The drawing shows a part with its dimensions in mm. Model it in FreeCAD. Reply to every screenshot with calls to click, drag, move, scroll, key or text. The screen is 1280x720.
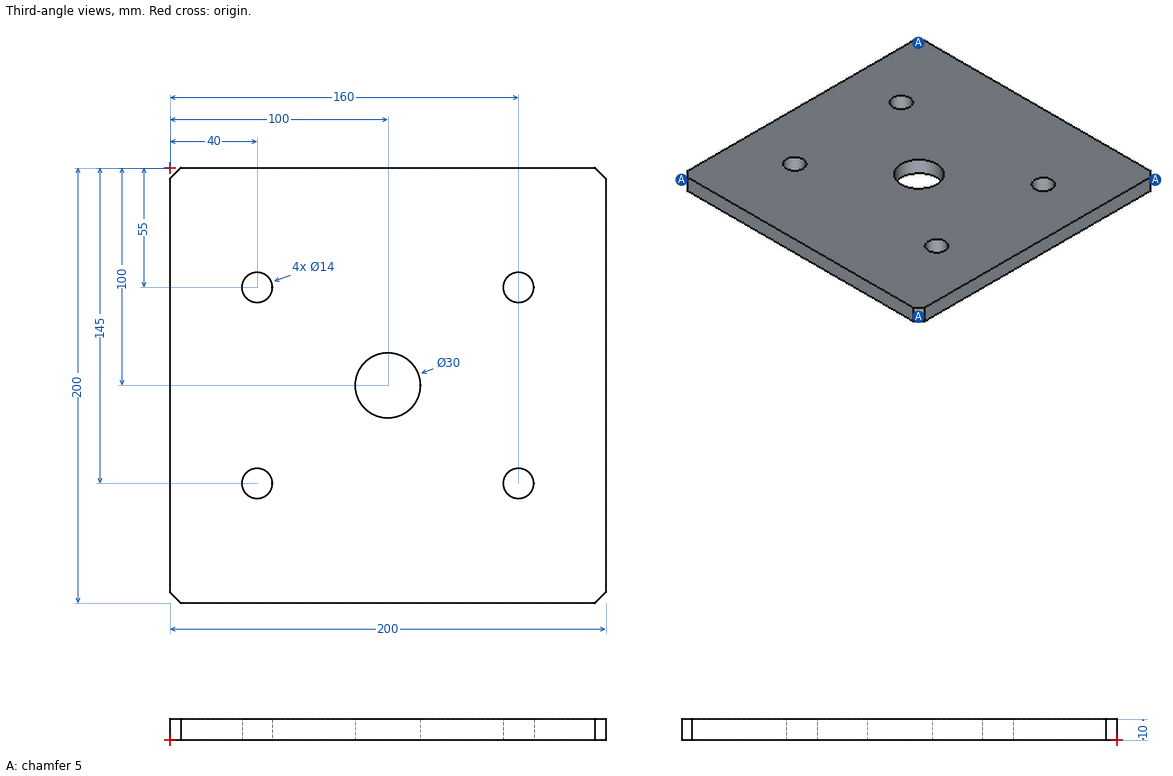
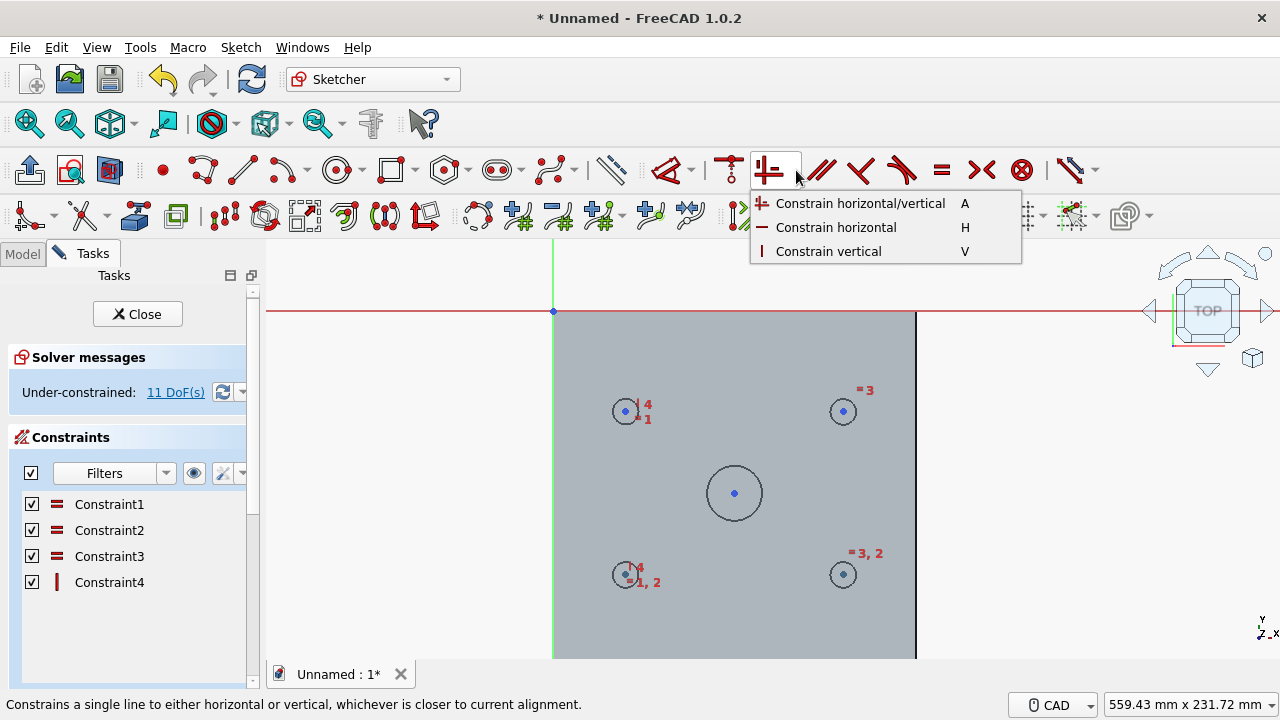
click(886, 227)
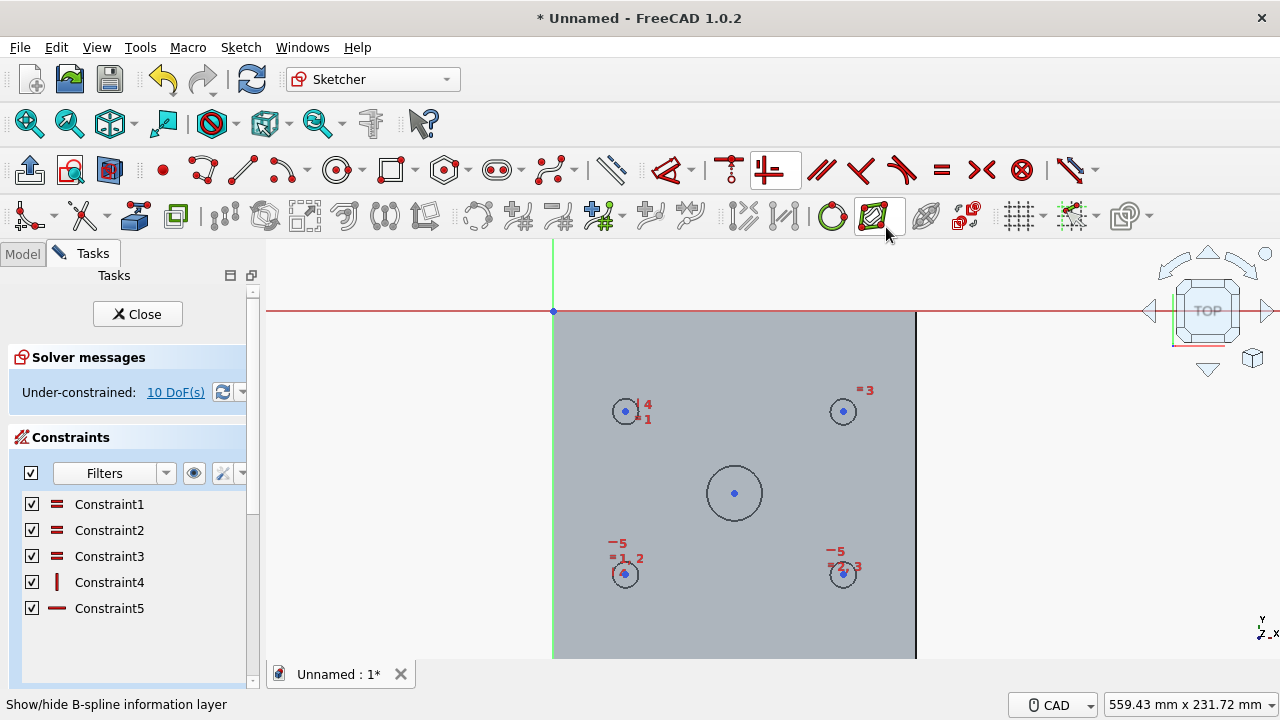
click(843, 575)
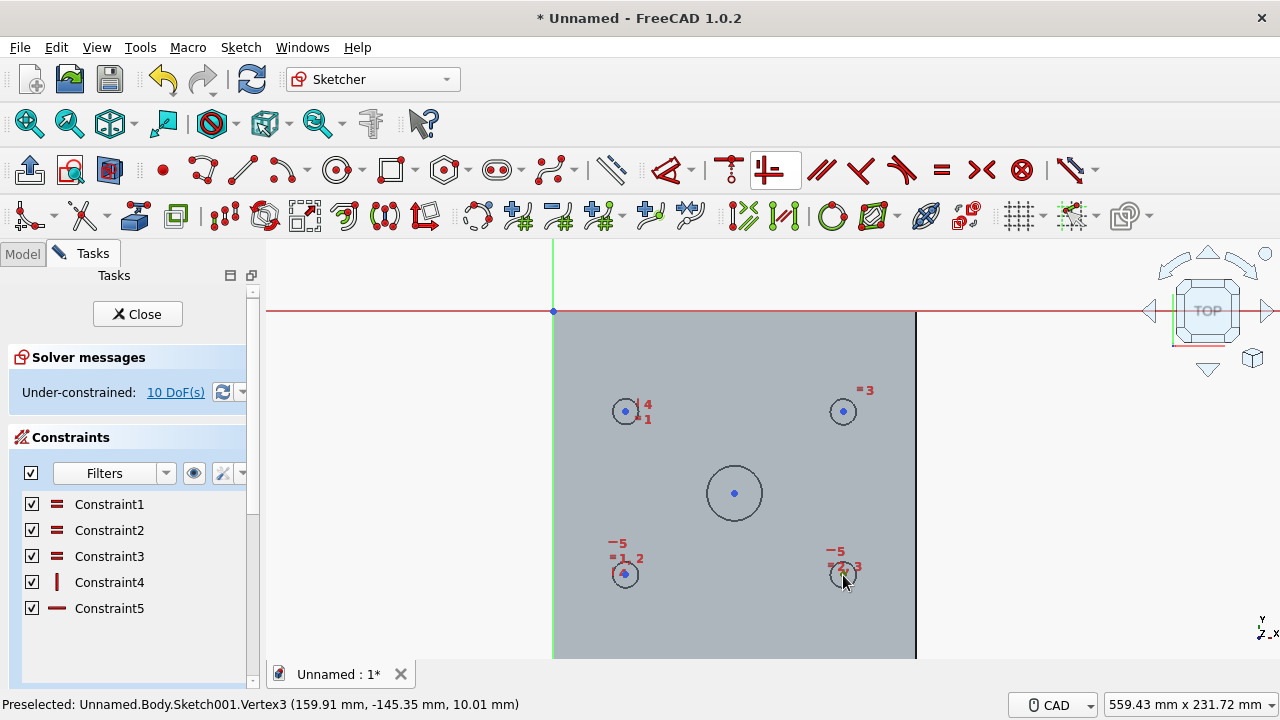
click(843, 412)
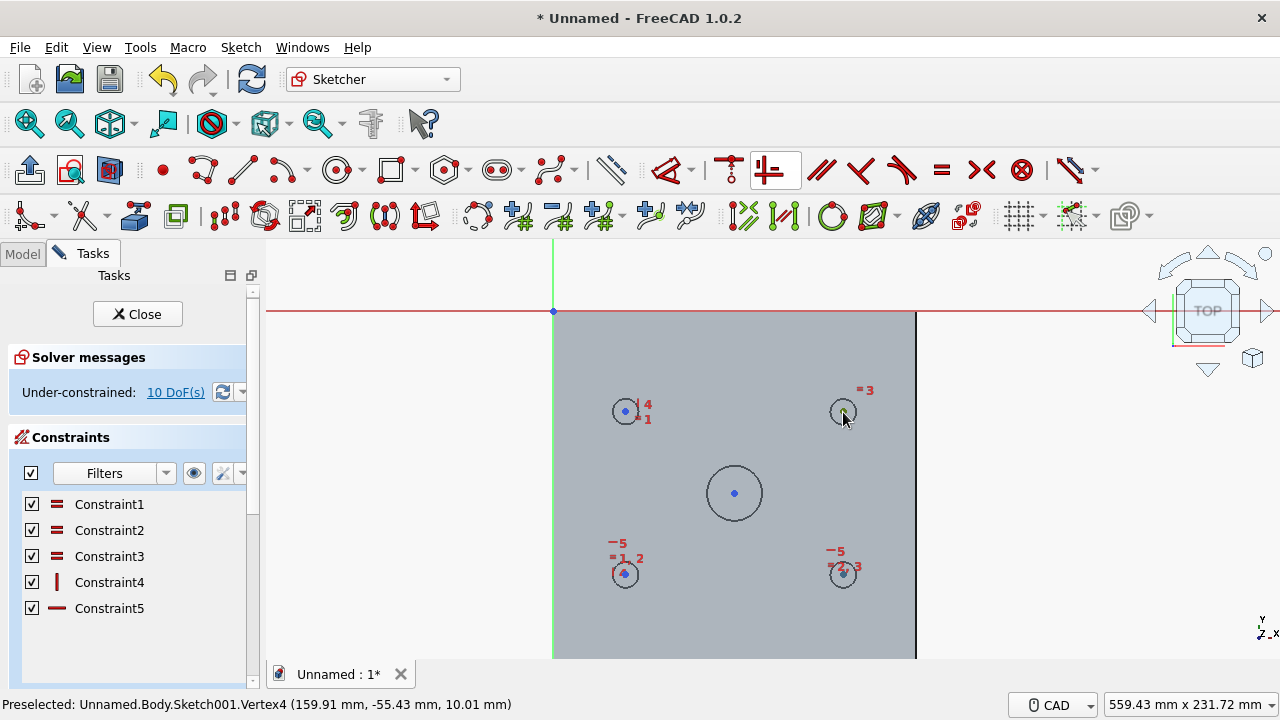
key(v)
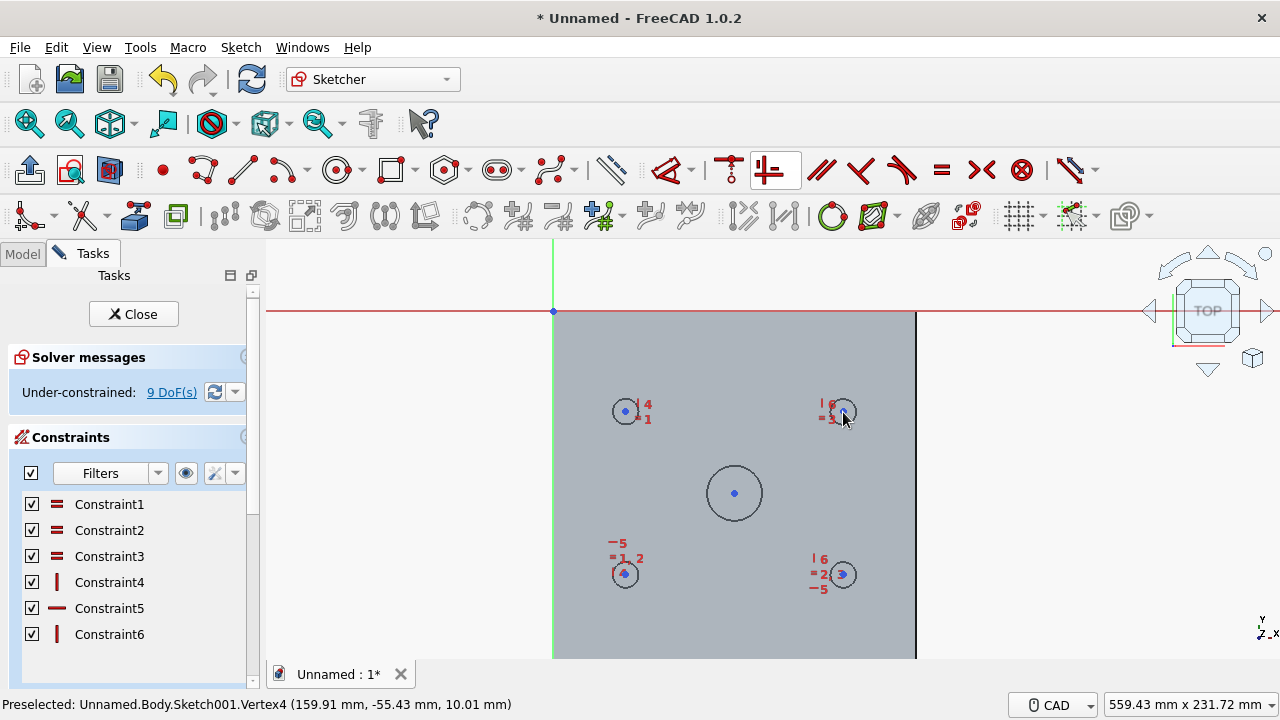
click(626, 412)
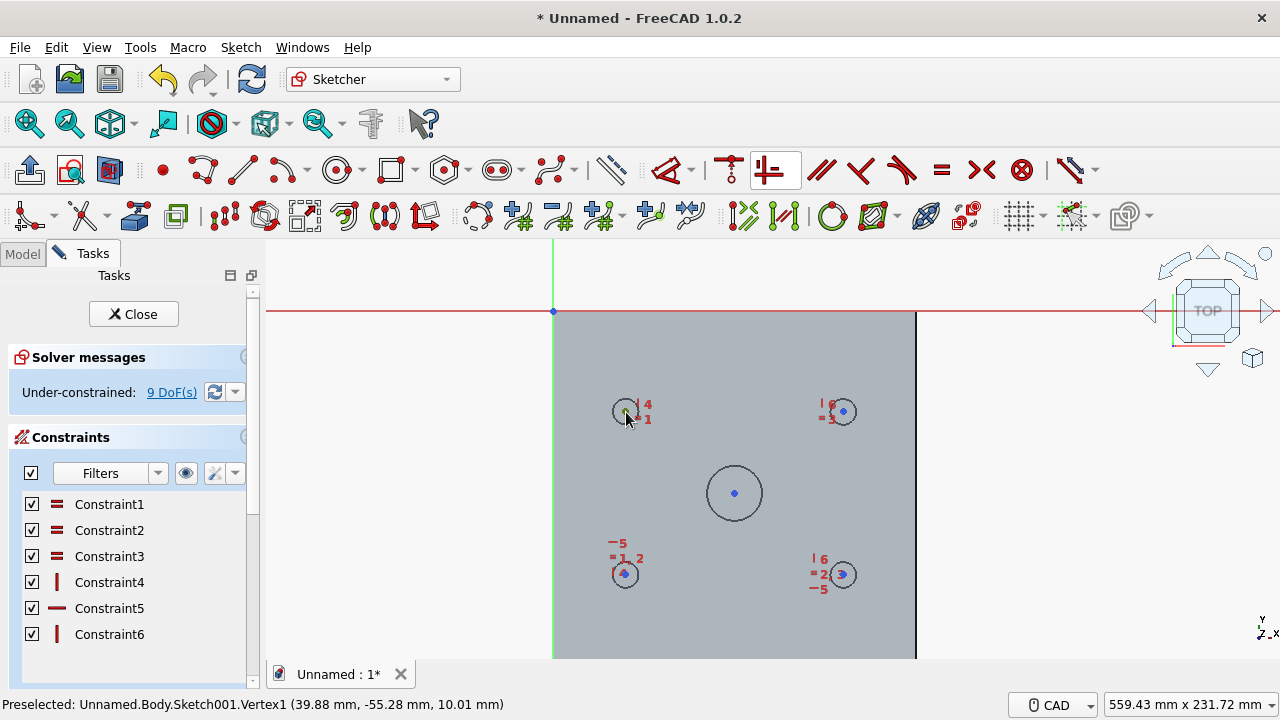
click(843, 412)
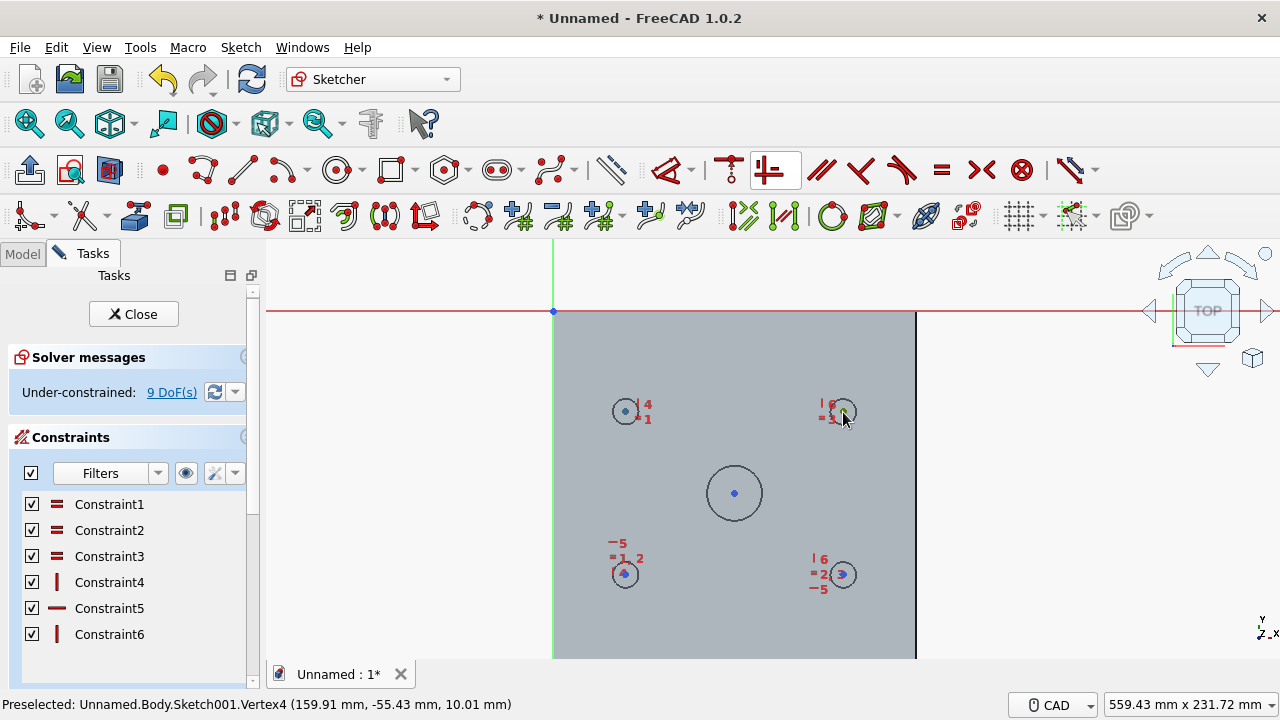
click(796, 170)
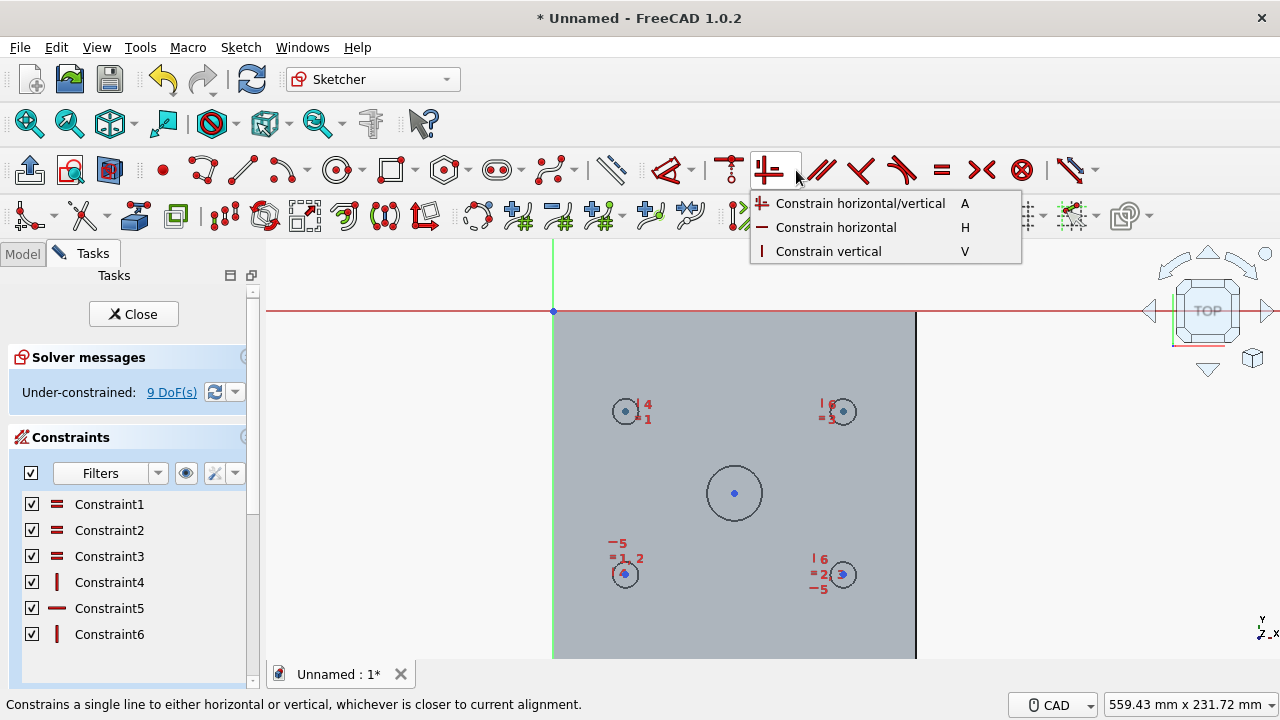
click(886, 227)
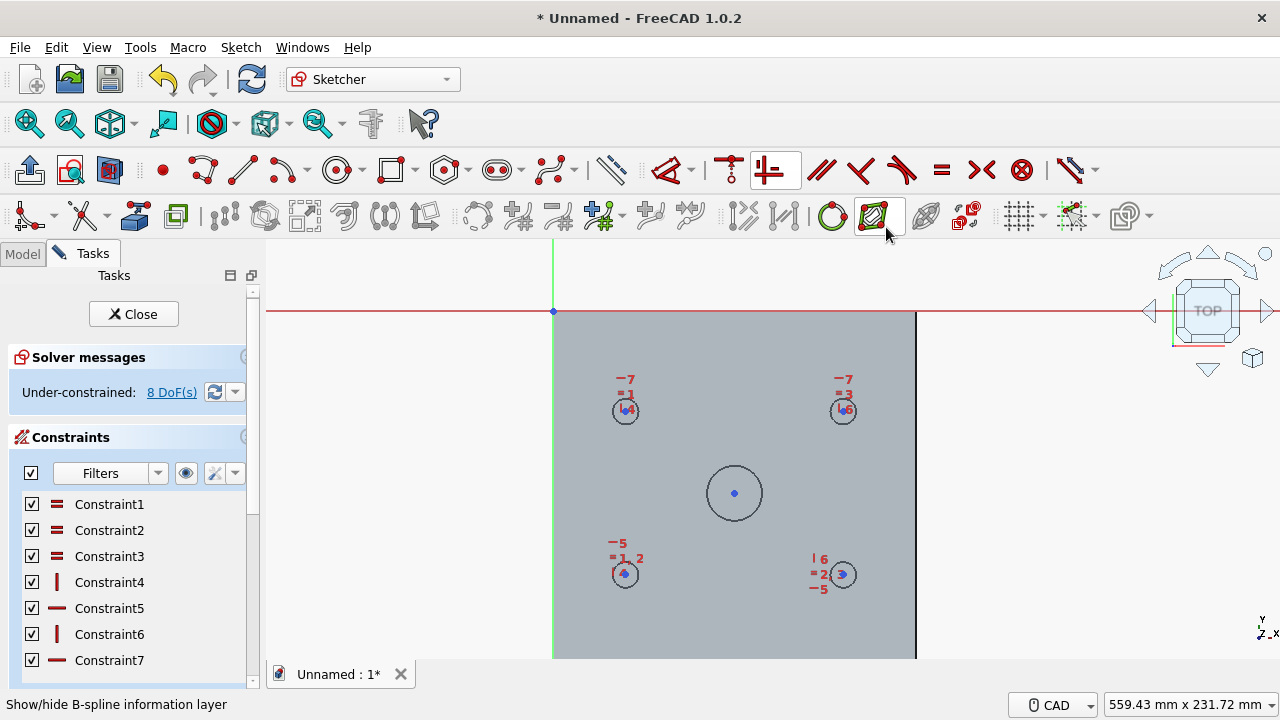
click(666, 170)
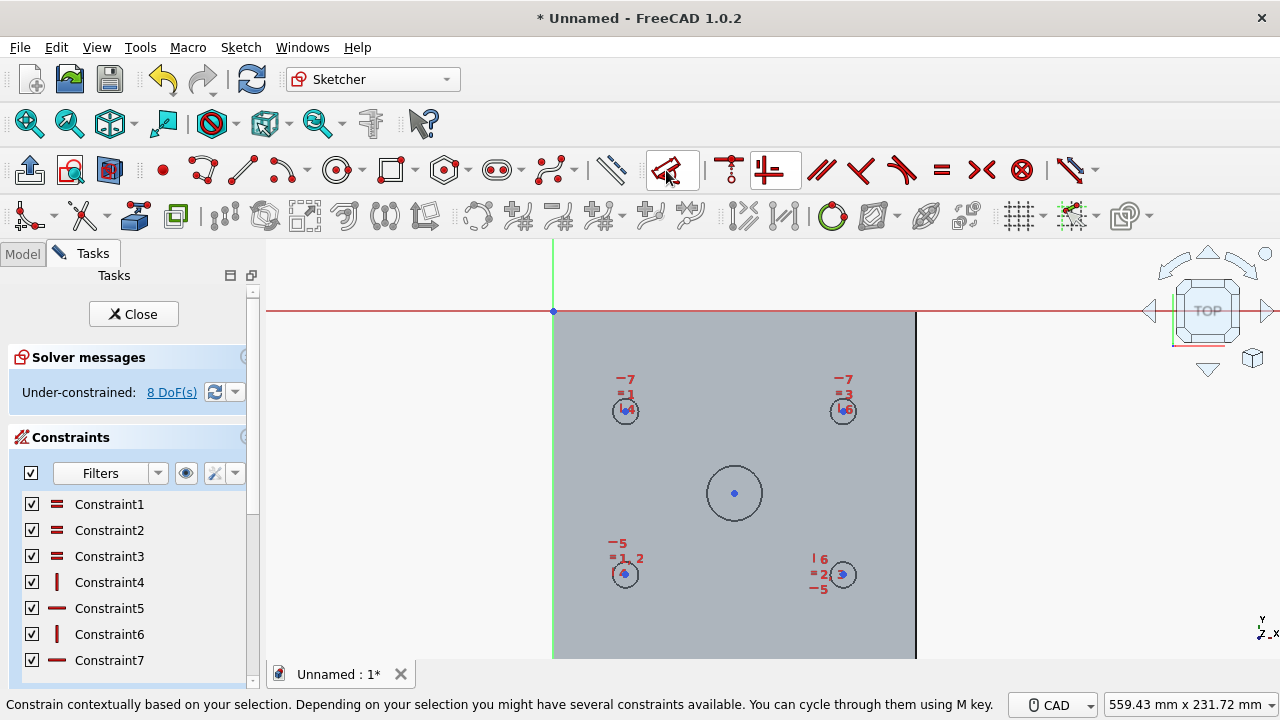
scroll(635, 403, up, 3)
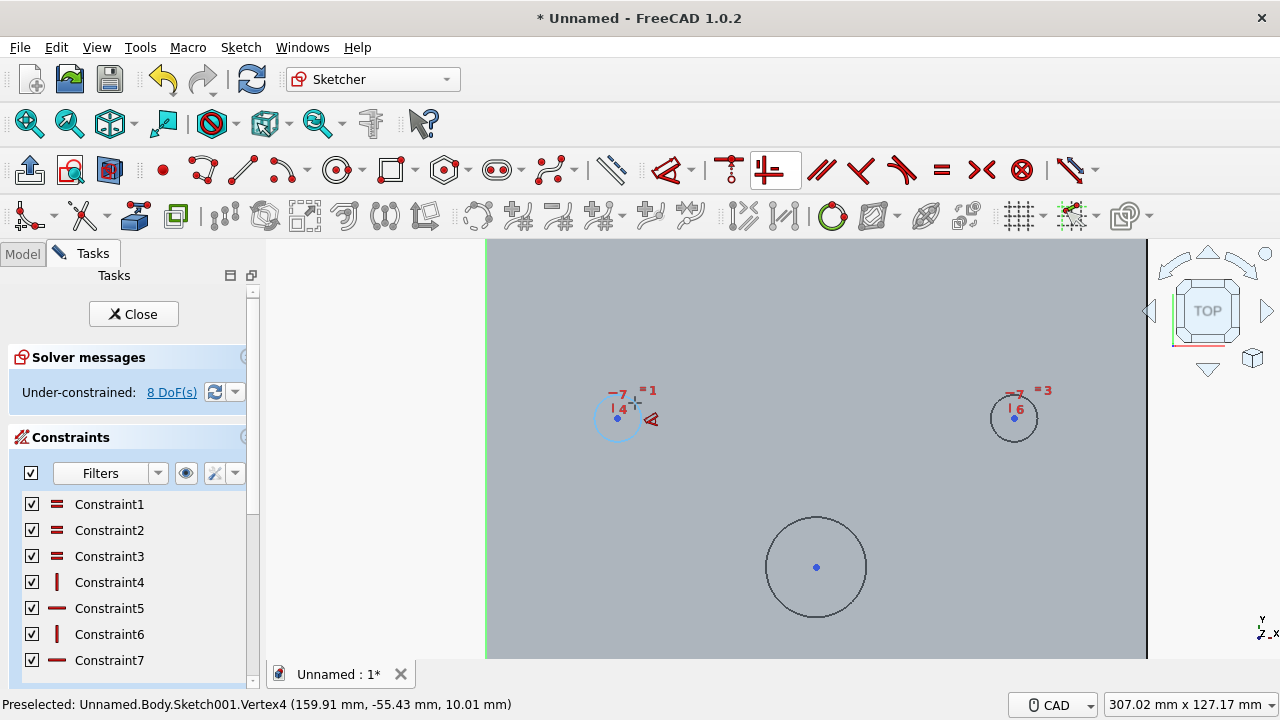
click(634, 402)
click(656, 379)